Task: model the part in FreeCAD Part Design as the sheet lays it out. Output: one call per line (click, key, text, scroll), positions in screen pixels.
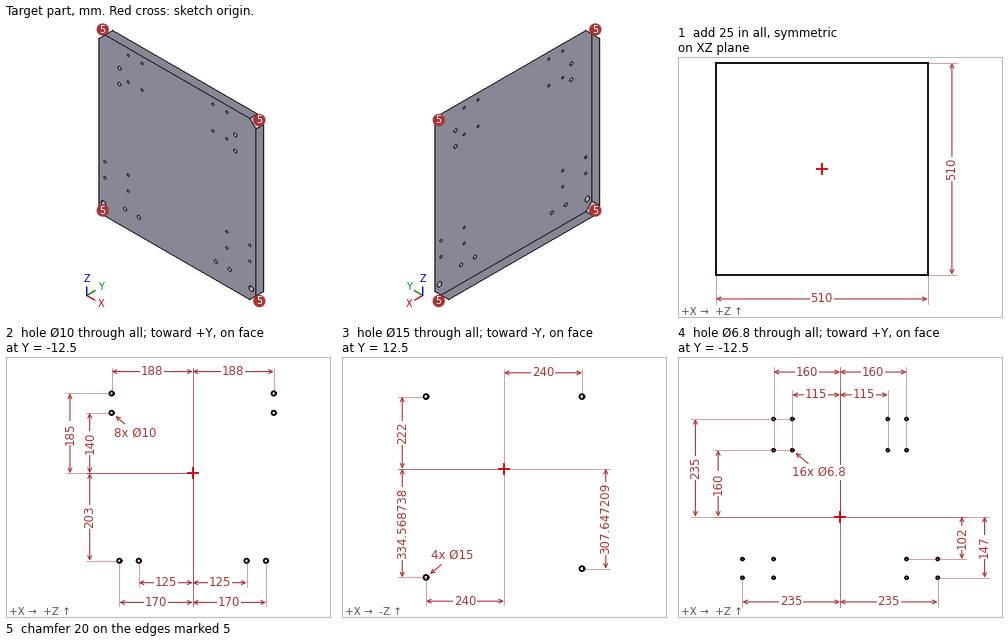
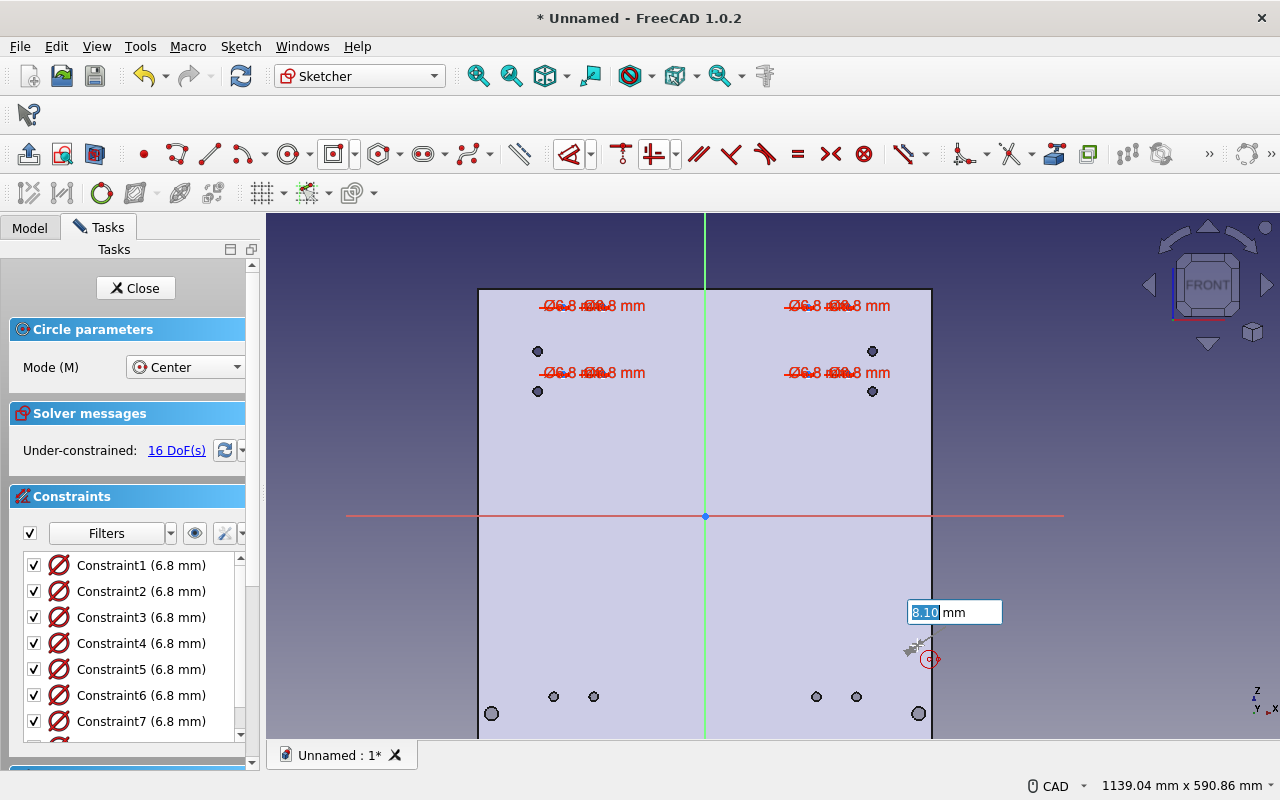
text(6.8)
key(Return)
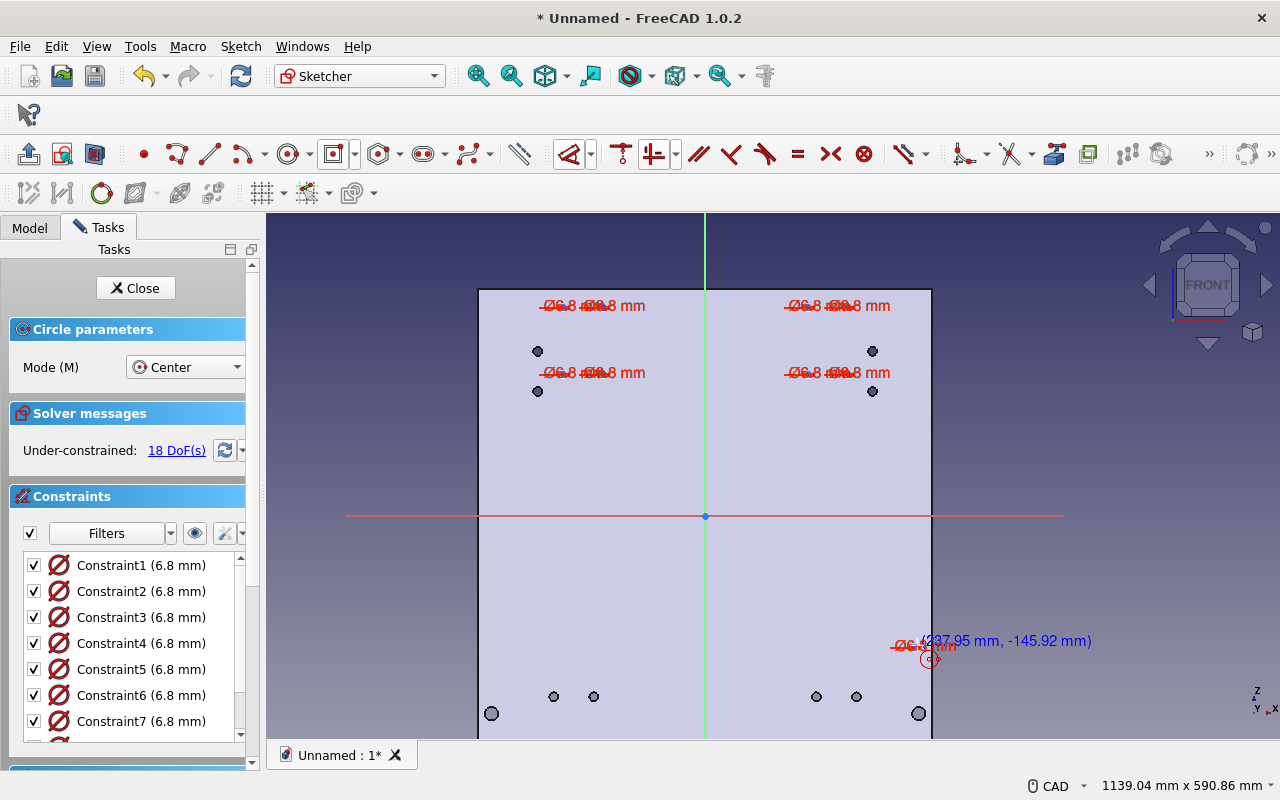
scroll(848, 647, up, 11)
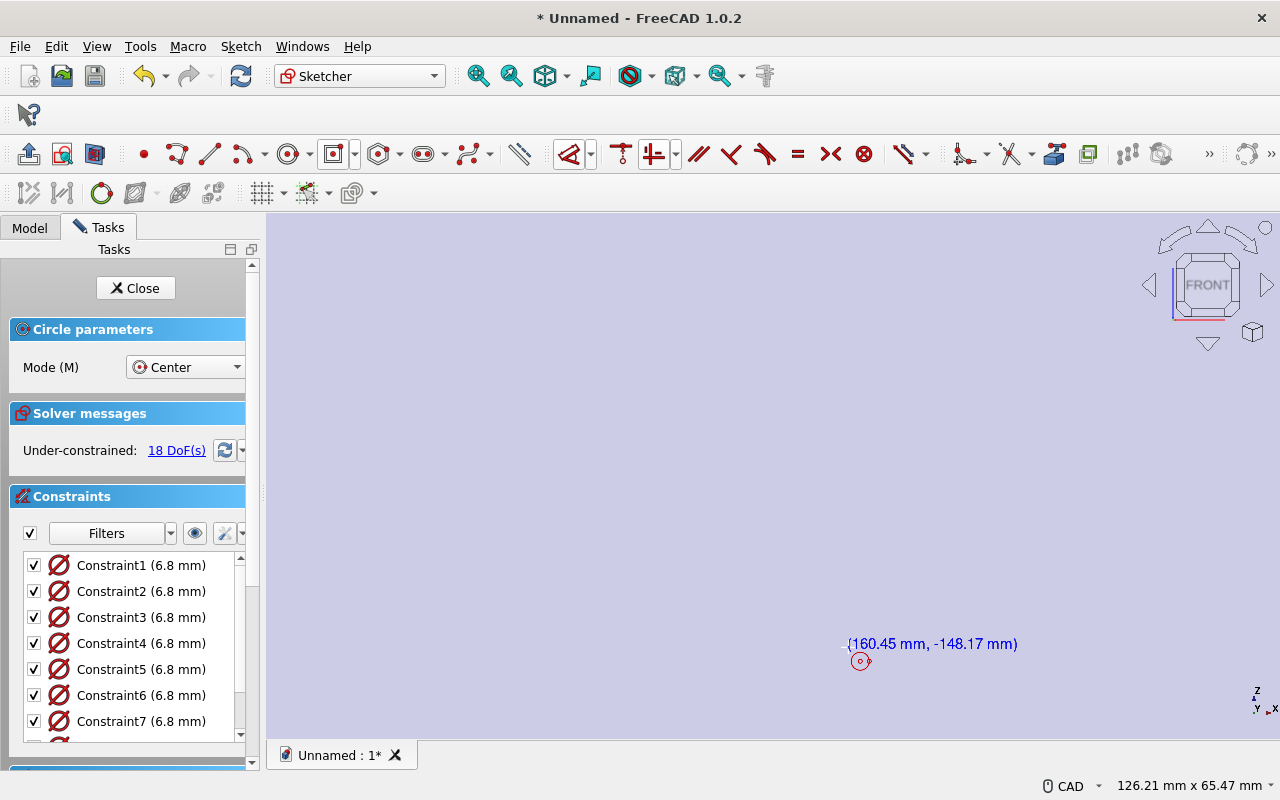
scroll(848, 647, down, 11)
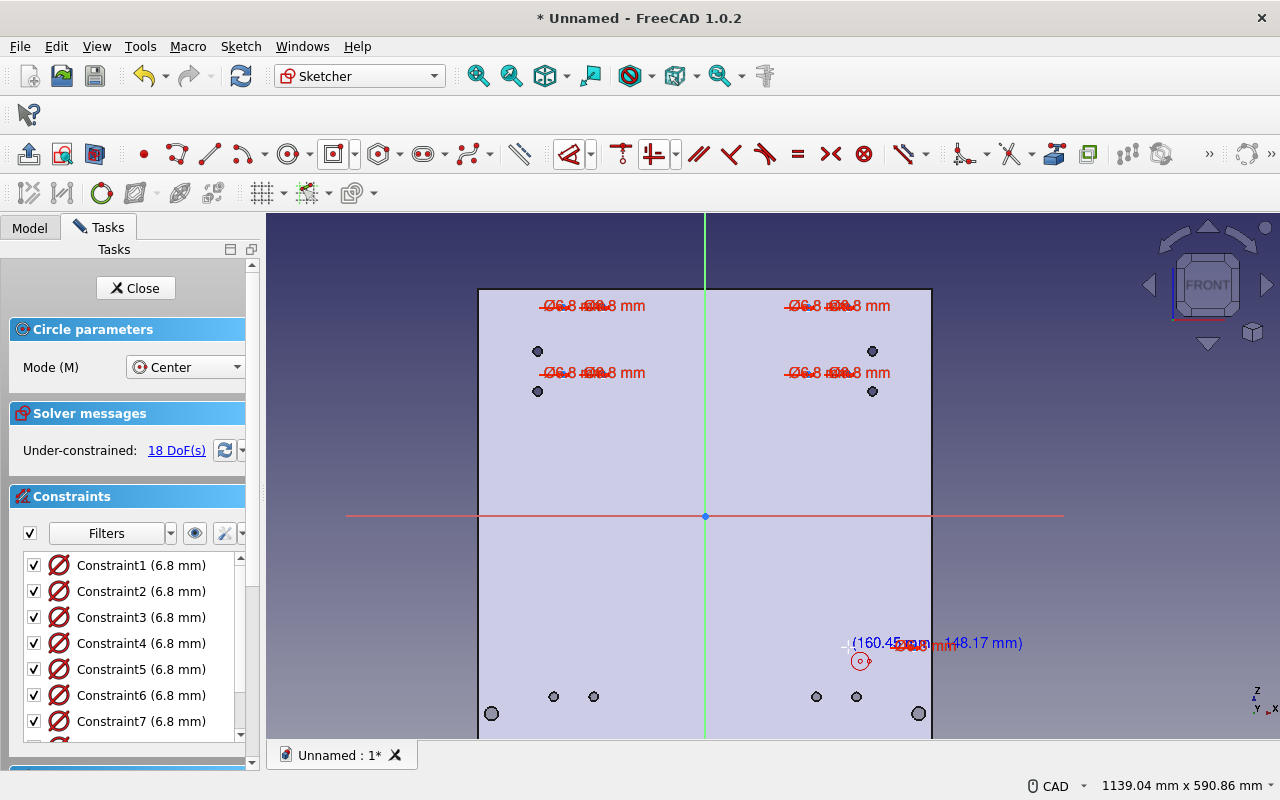
click(848, 647)
move(850, 645)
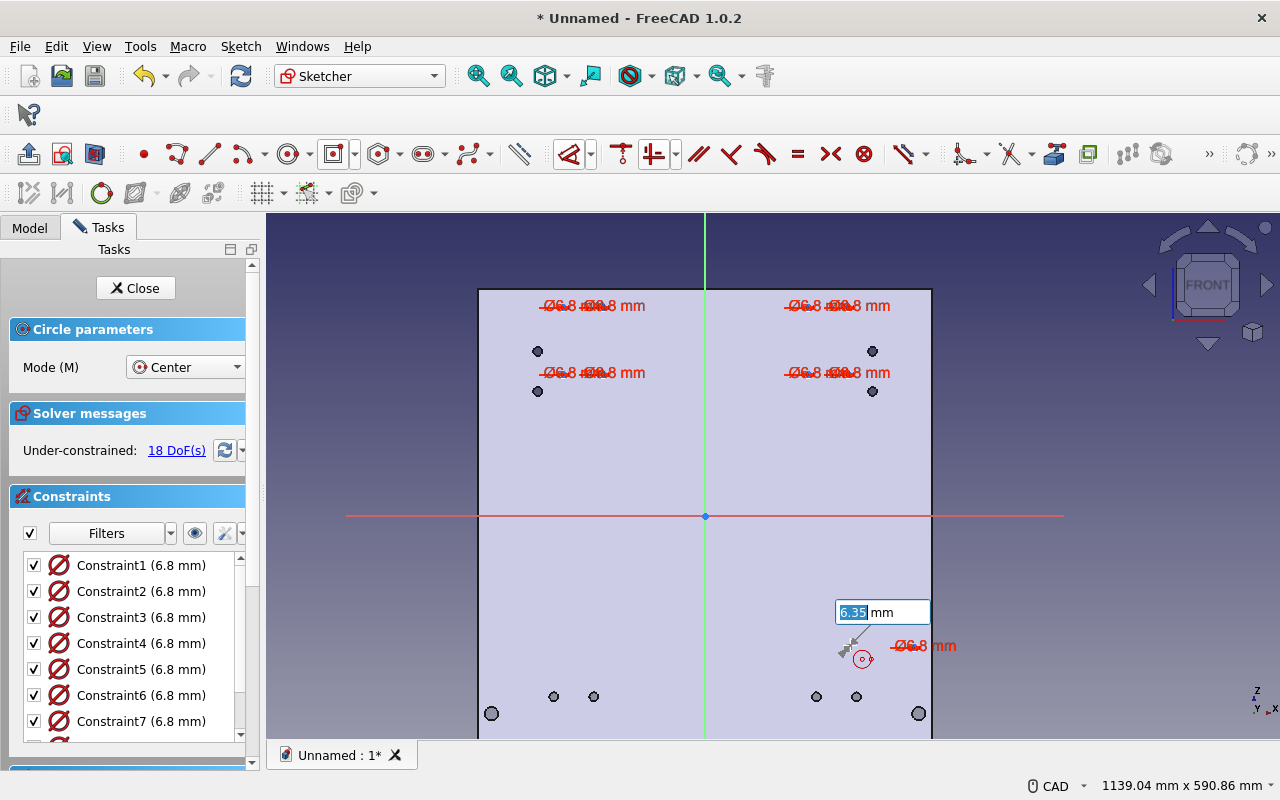
text(6.8)
key(Return)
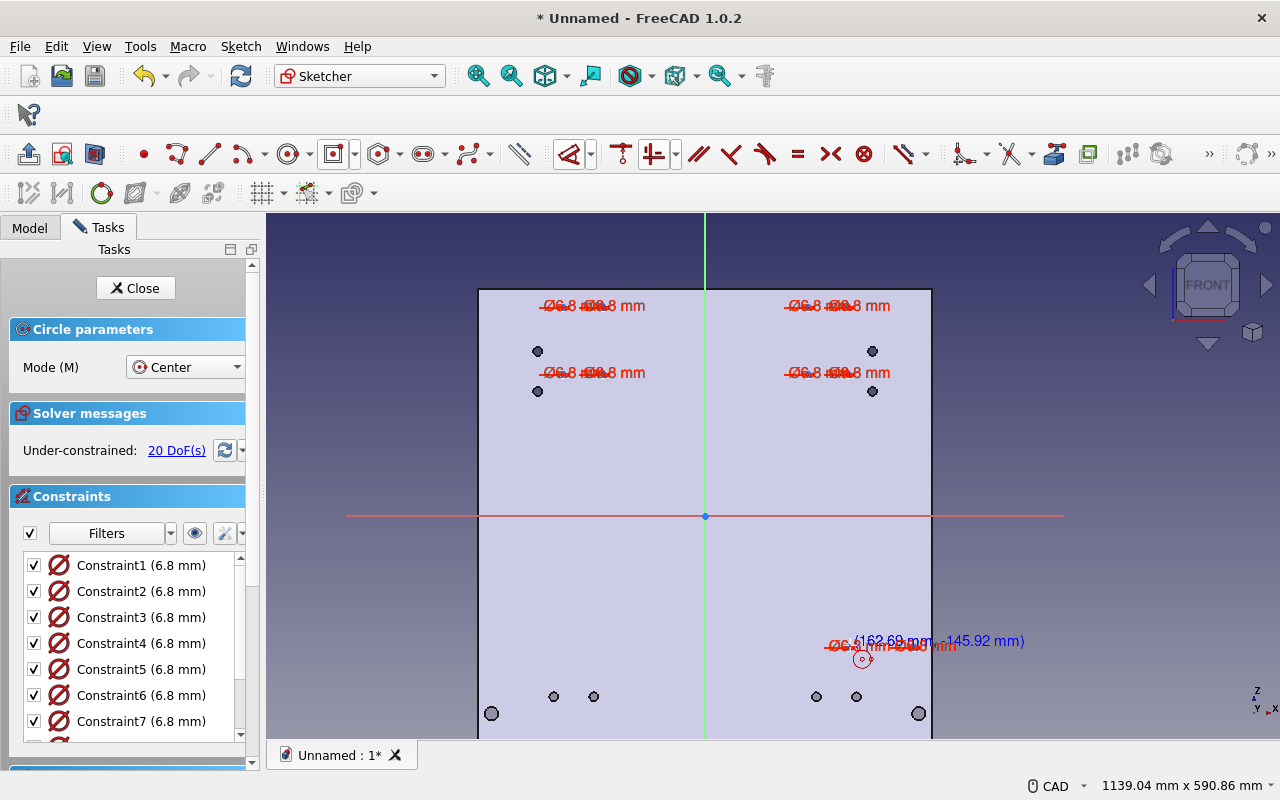
scroll(848, 607, up, 11)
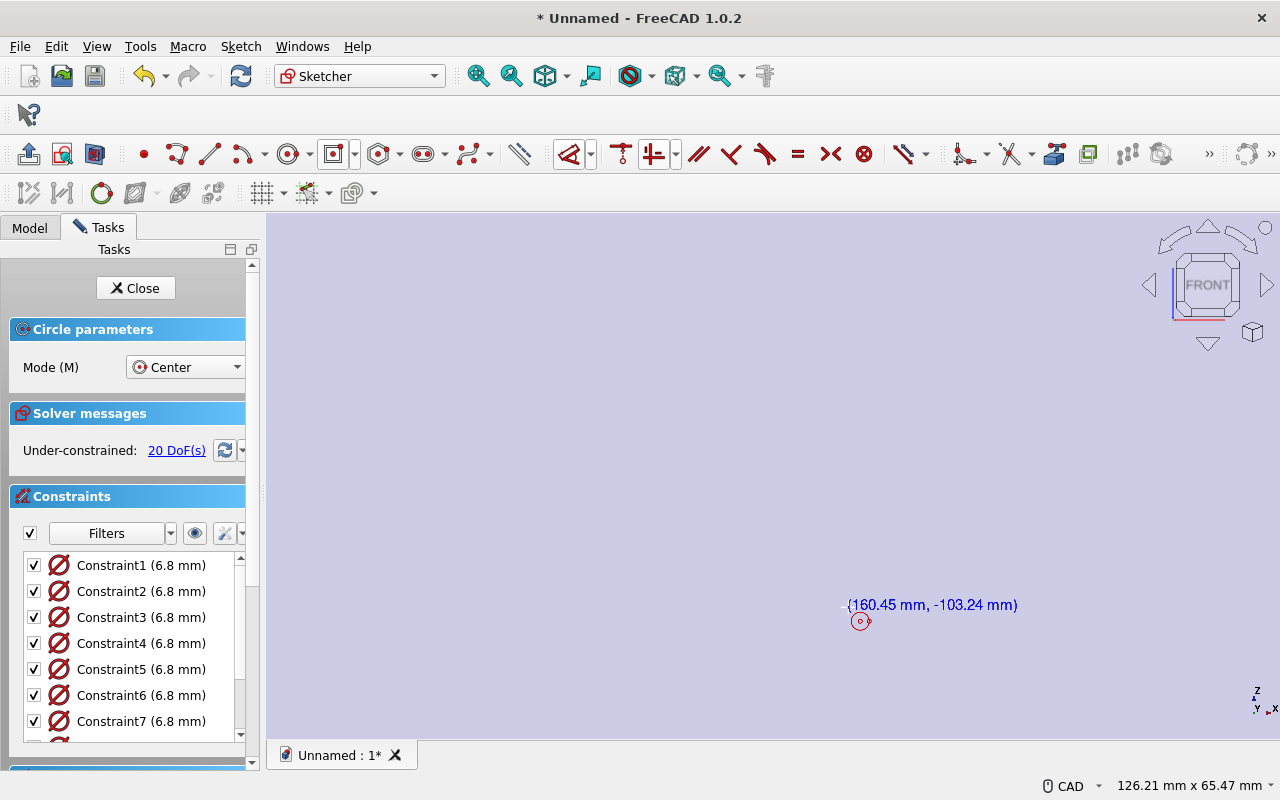
scroll(848, 607, down, 11)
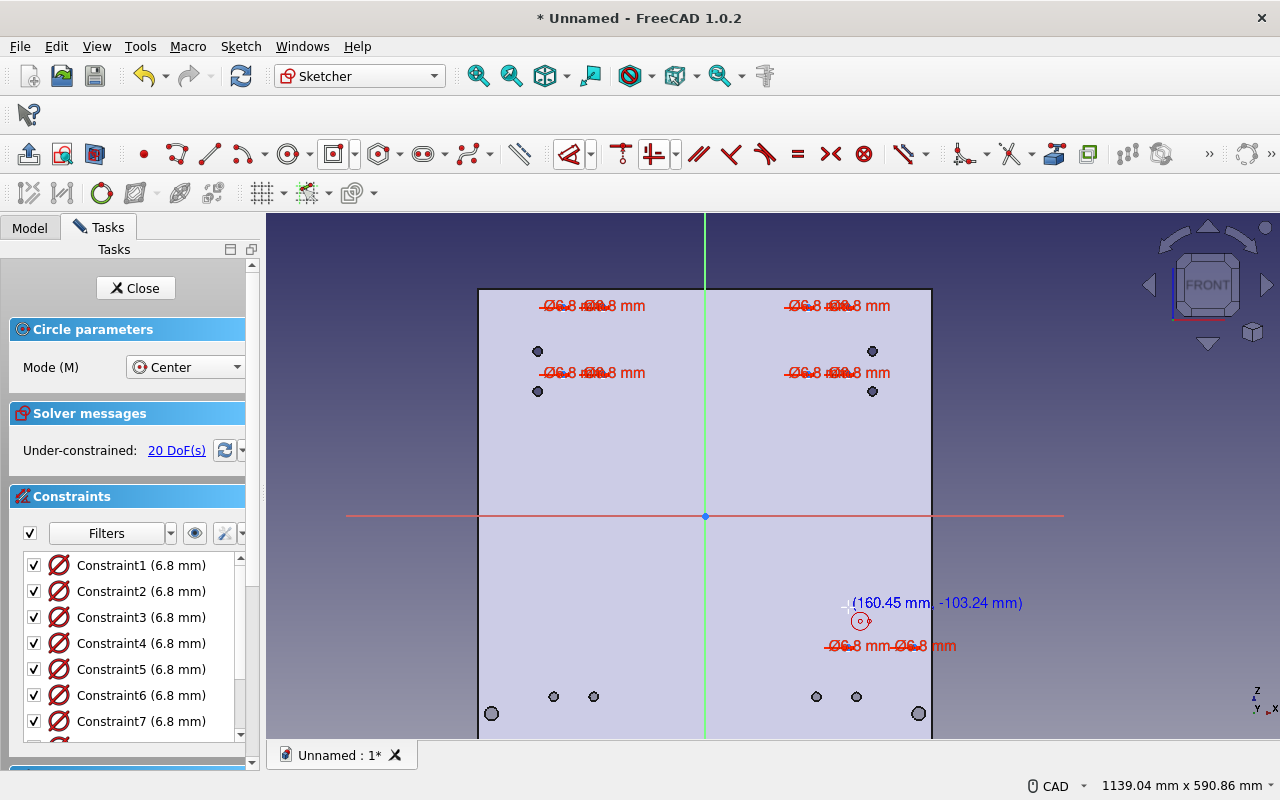
click(848, 607)
move(850, 605)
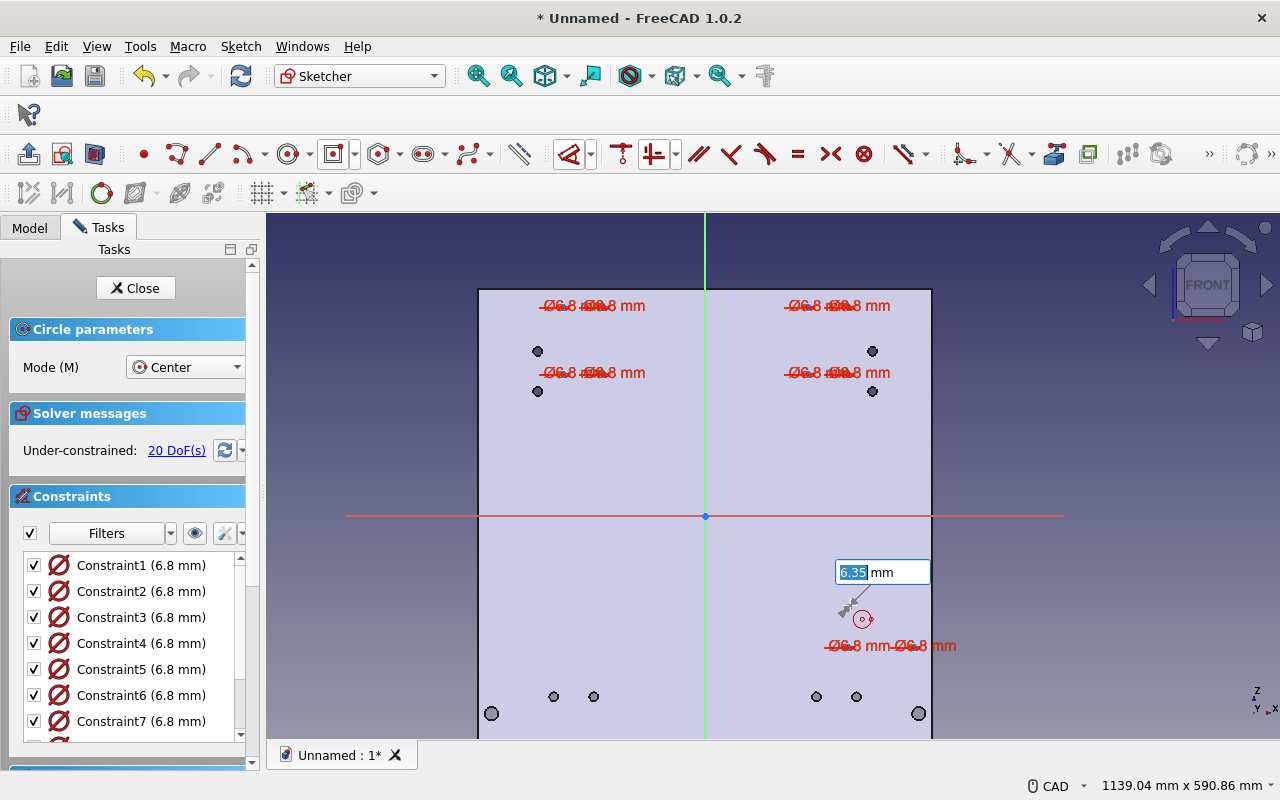
text(6.8)
key(Return)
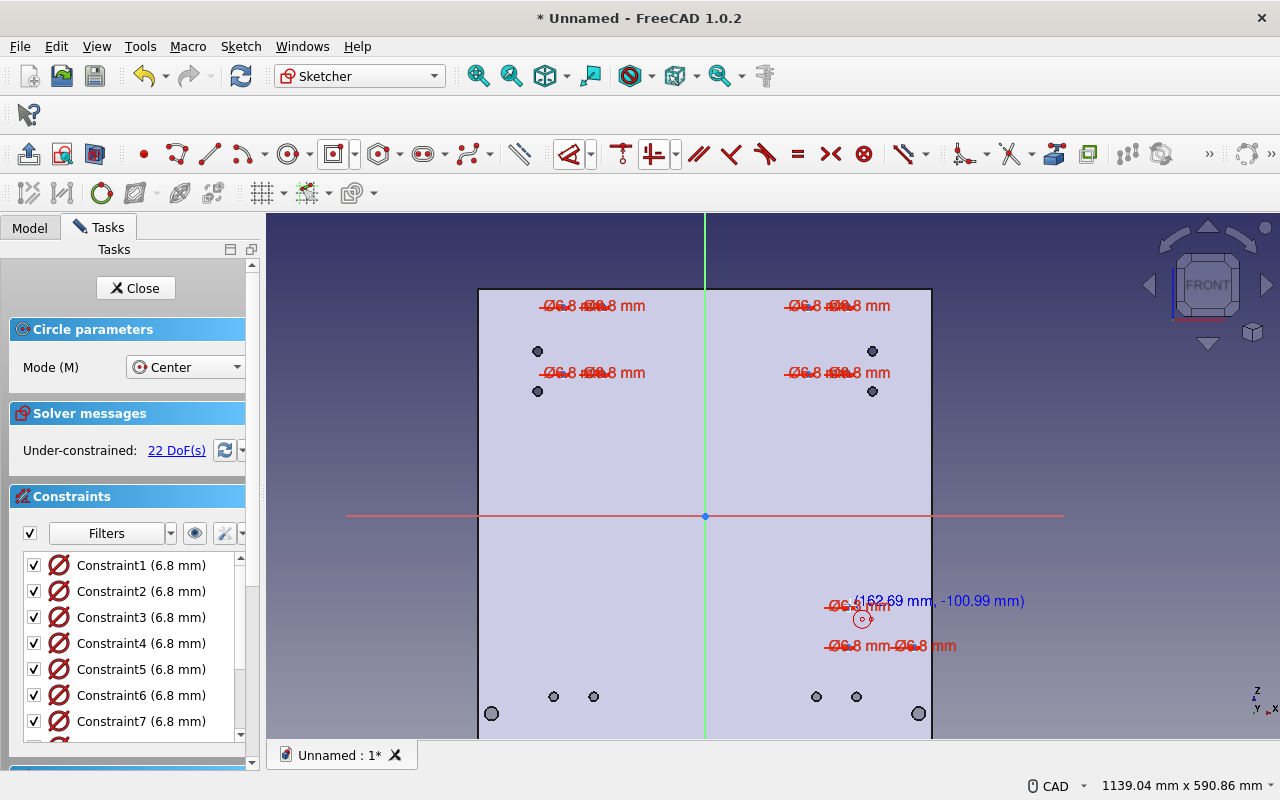
scroll(914, 607, up, 11)